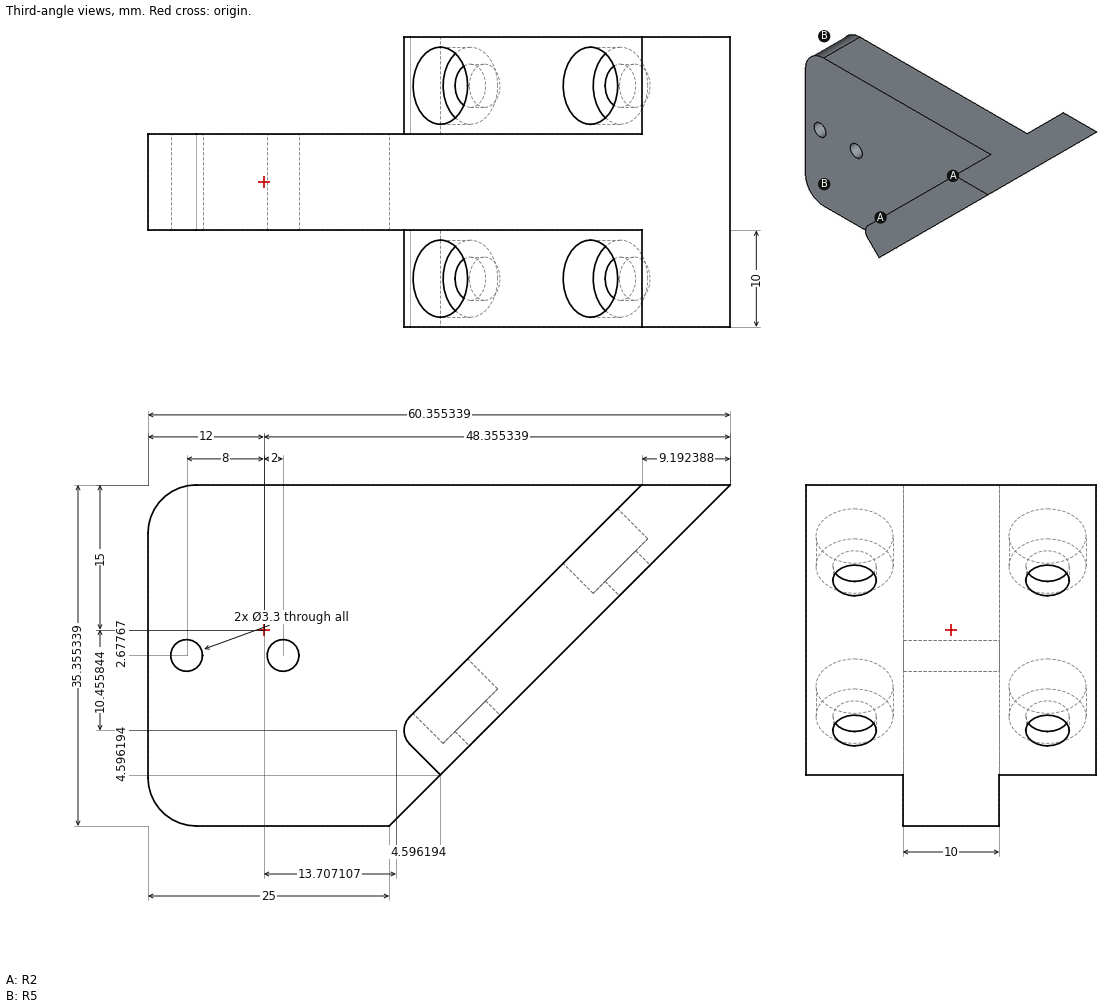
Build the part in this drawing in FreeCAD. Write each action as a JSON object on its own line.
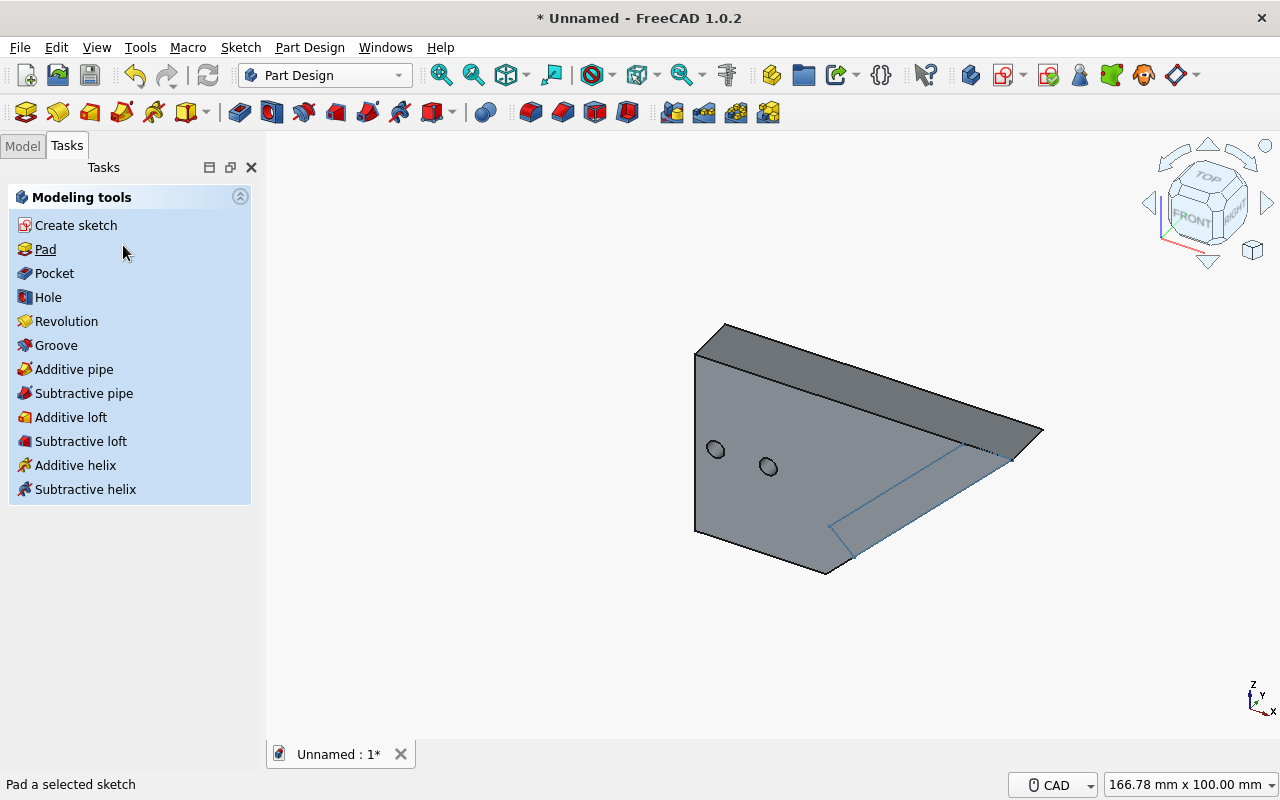
{"action": "left_click", "coordinate": [26, 112]}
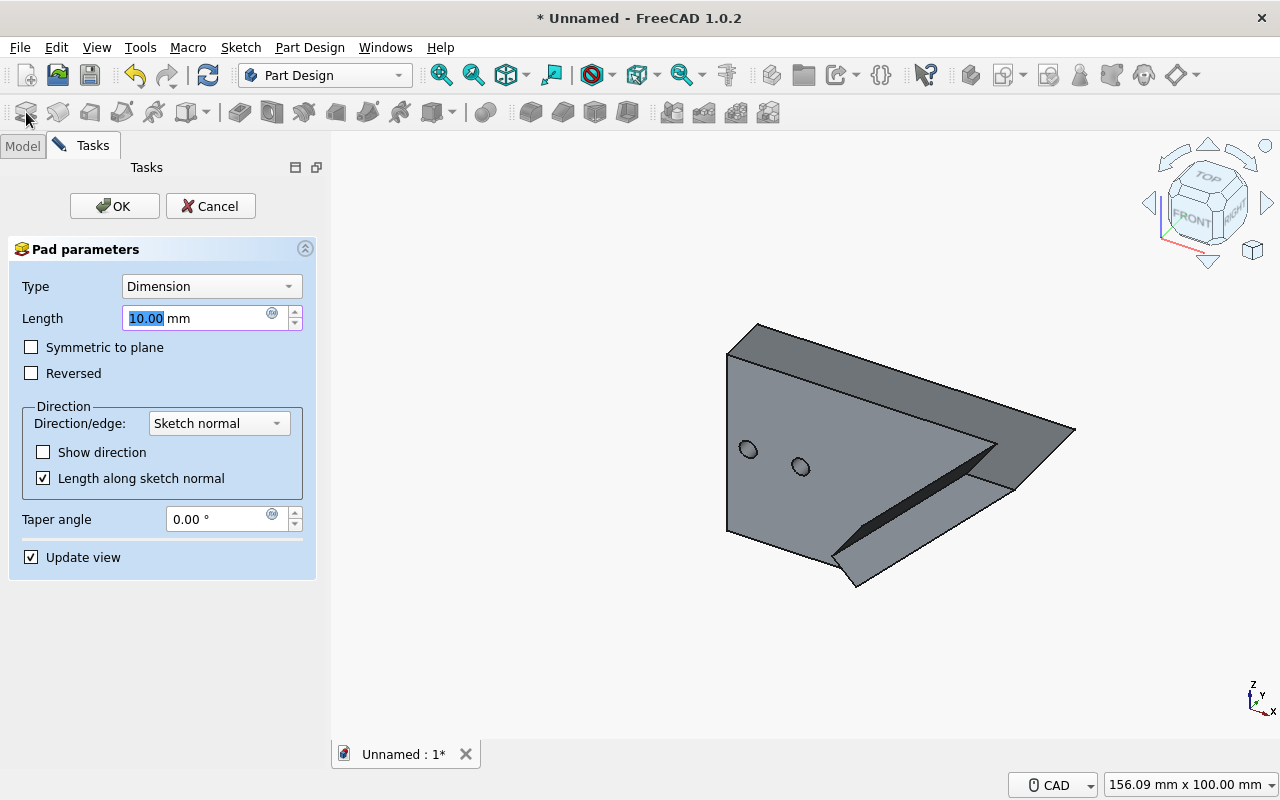
{"action": "type", "text": "10"}
{"action": "key", "text": "Tab"}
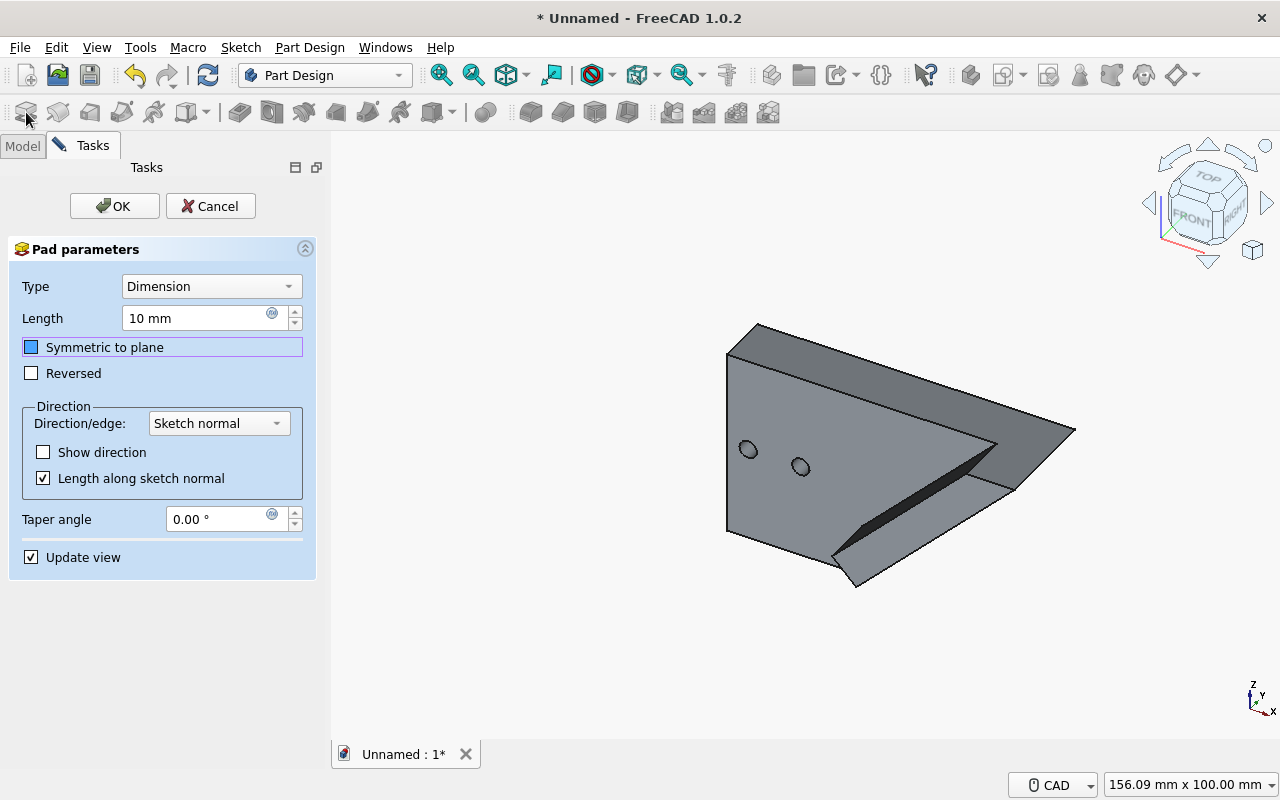
{"action": "left_click", "coordinate": [115, 206]}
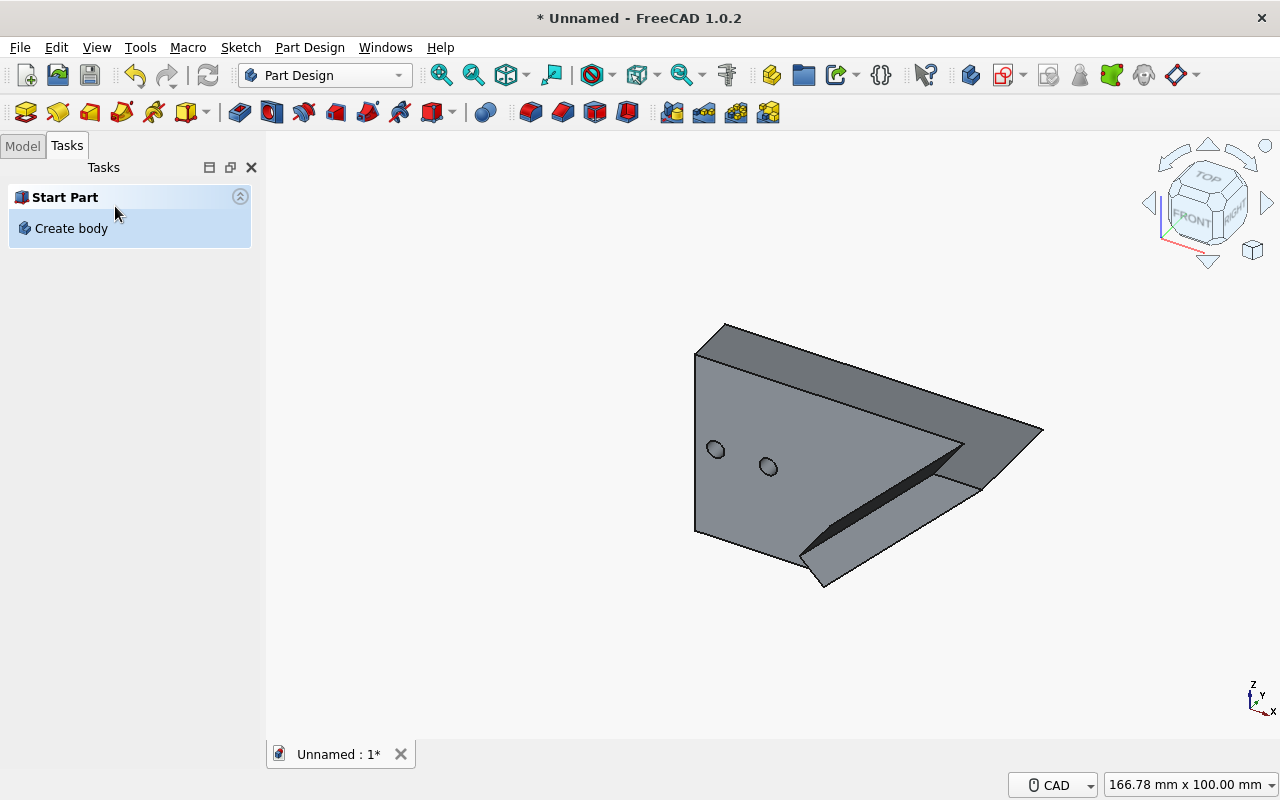
{"action": "left_click", "coordinate": [23, 145]}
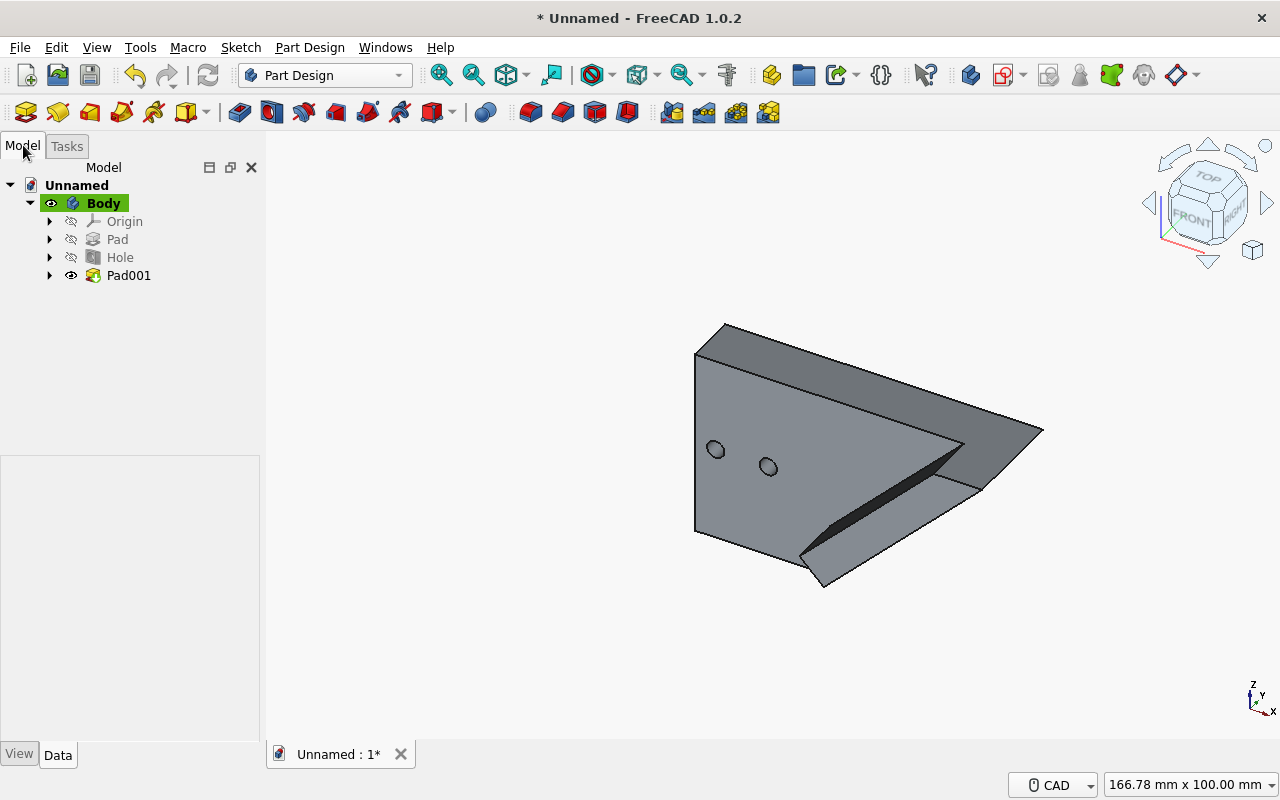
{"action": "left_click", "coordinate": [116, 275]}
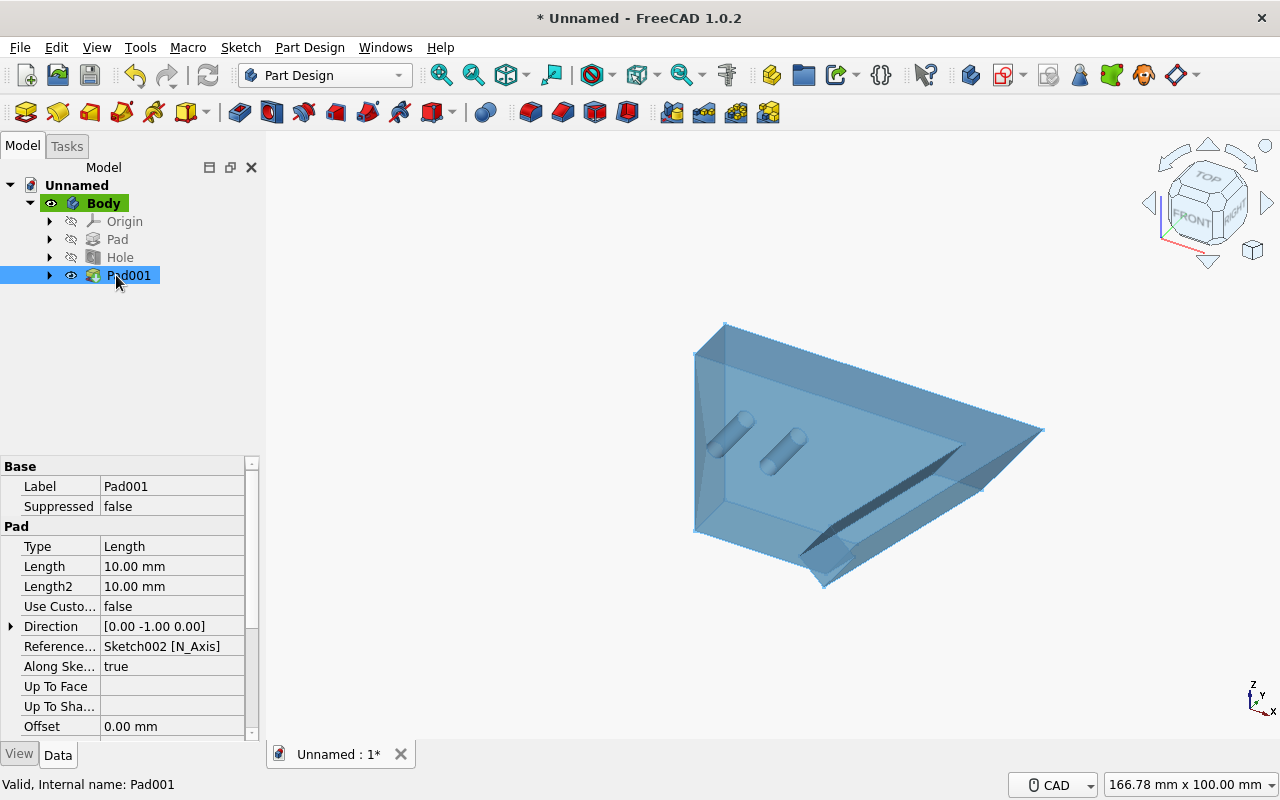
{"action": "left_click", "coordinate": [672, 112]}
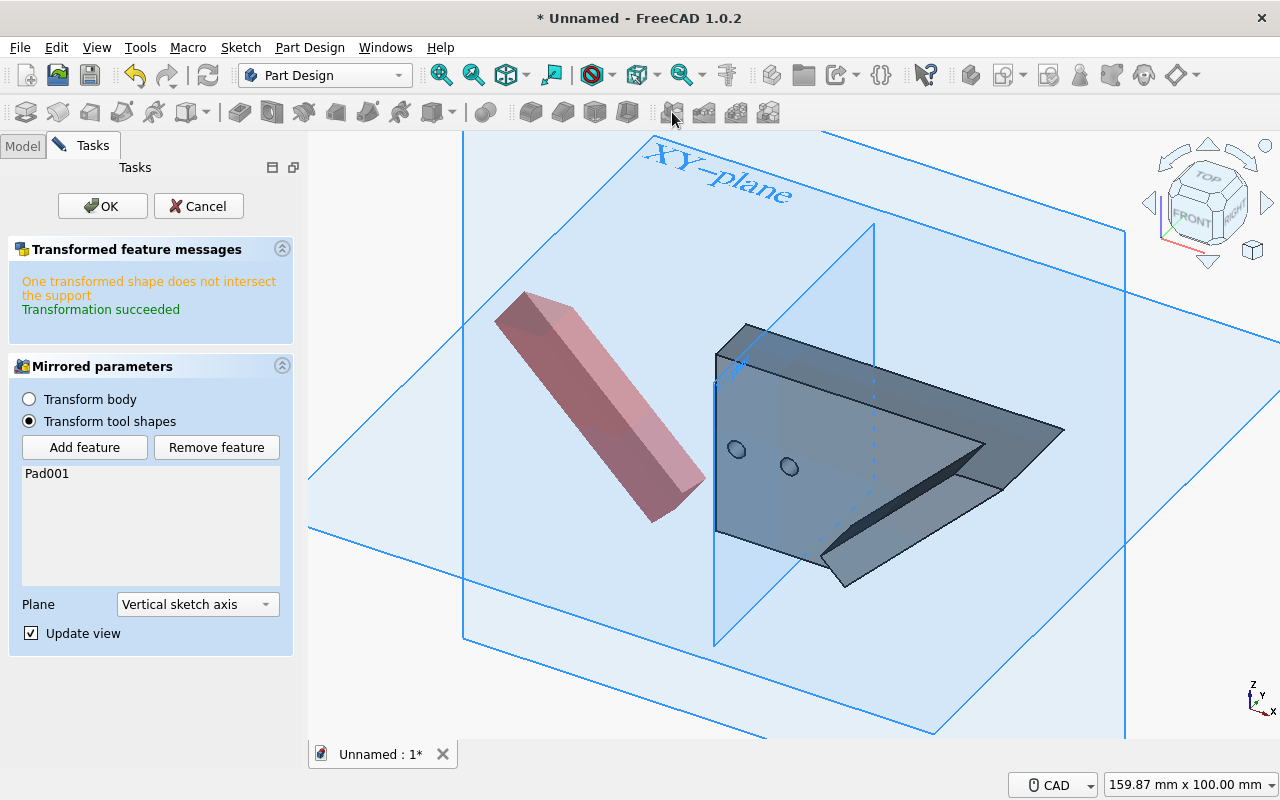
{"action": "left_click", "coordinate": [198, 604]}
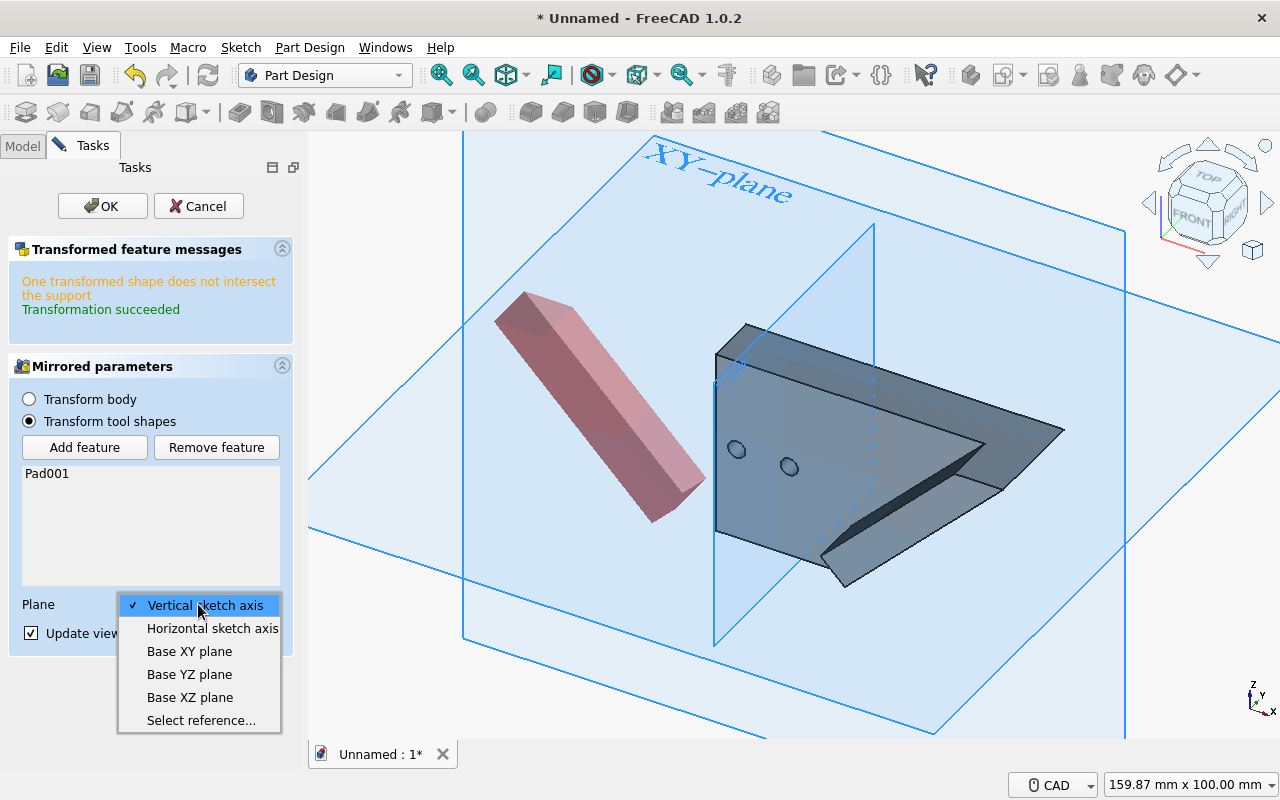
{"action": "left_click", "coordinate": [198, 698]}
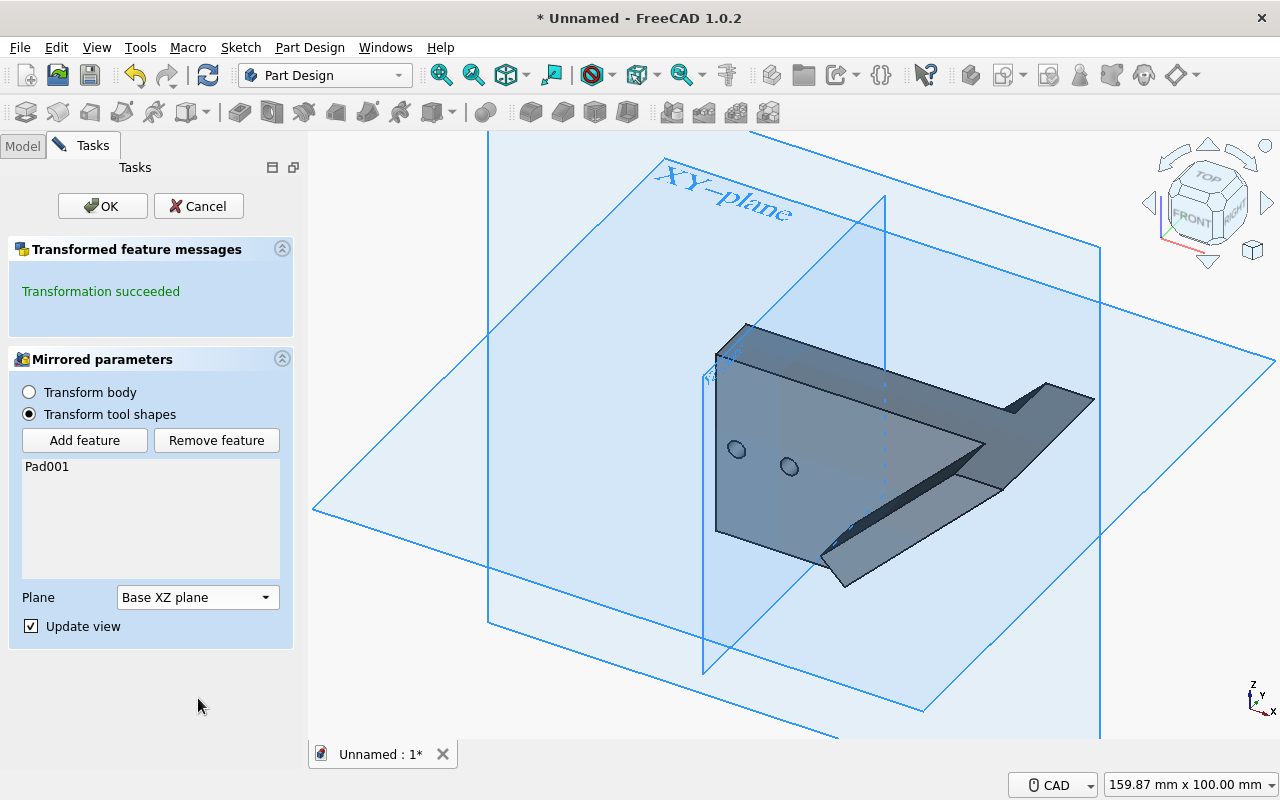
{"action": "left_click", "coordinate": [103, 206]}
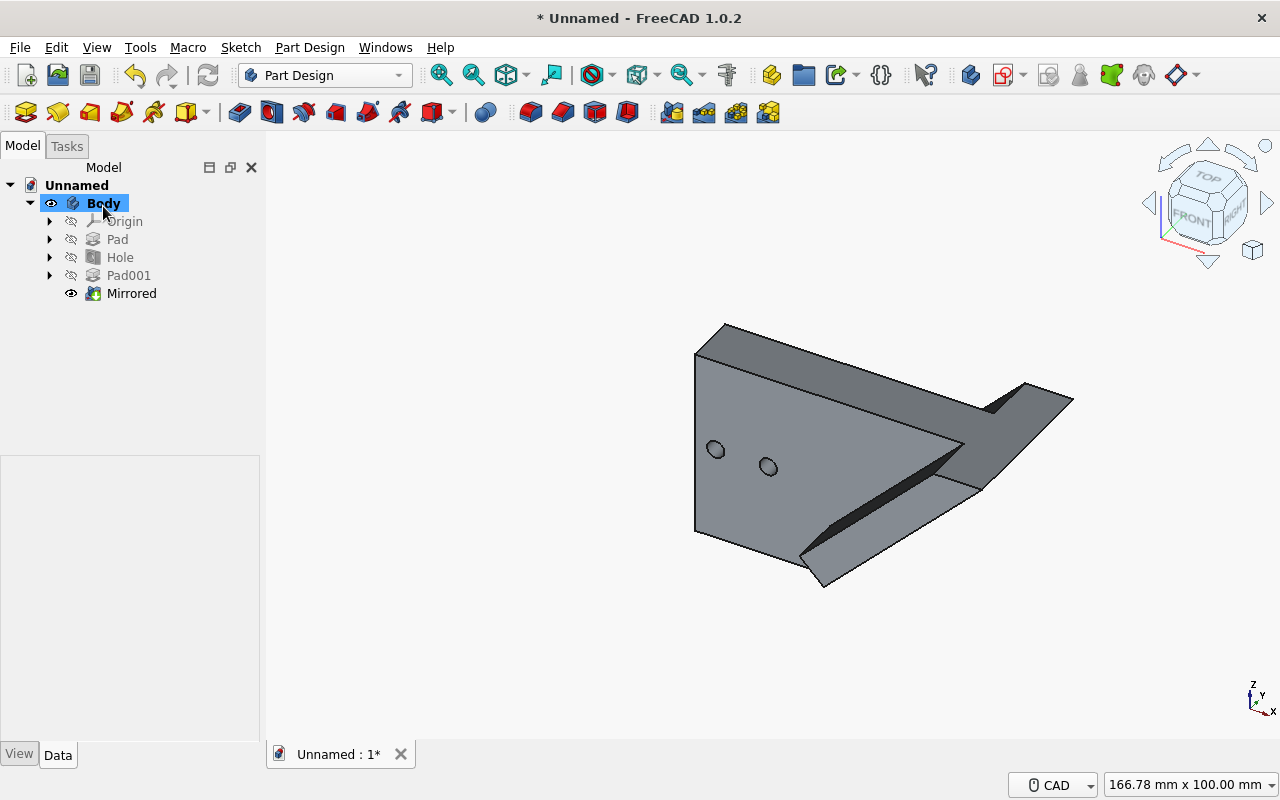
{"action": "key", "text": "2"}